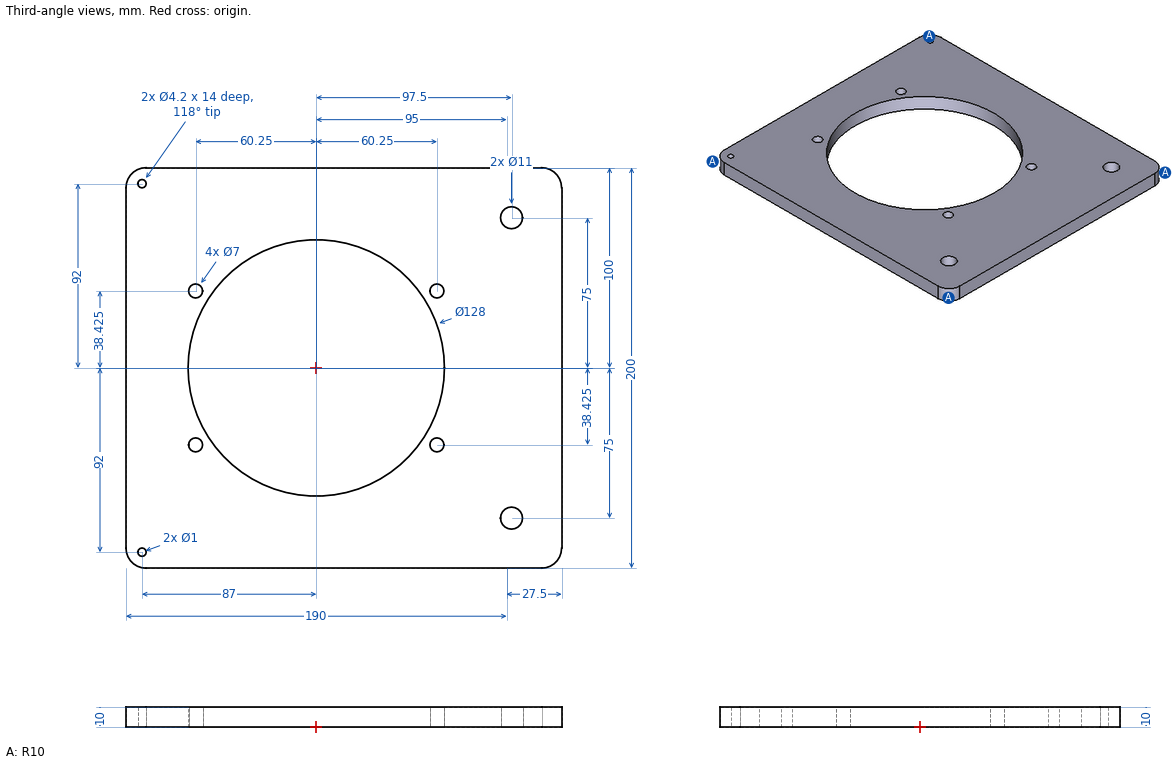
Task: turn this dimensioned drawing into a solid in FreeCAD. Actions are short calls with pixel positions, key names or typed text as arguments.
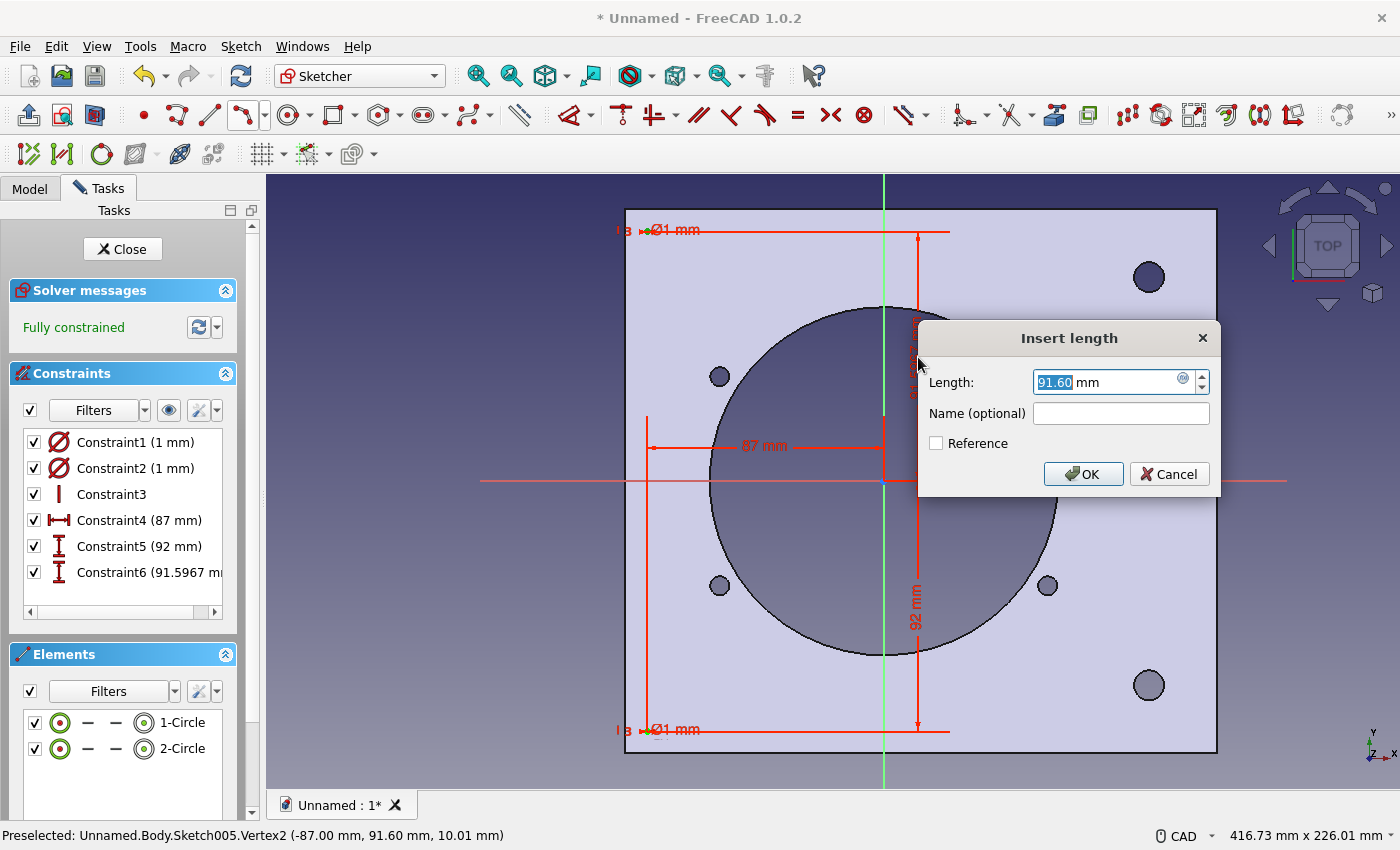
text(92)
key(Return)
key(Escape)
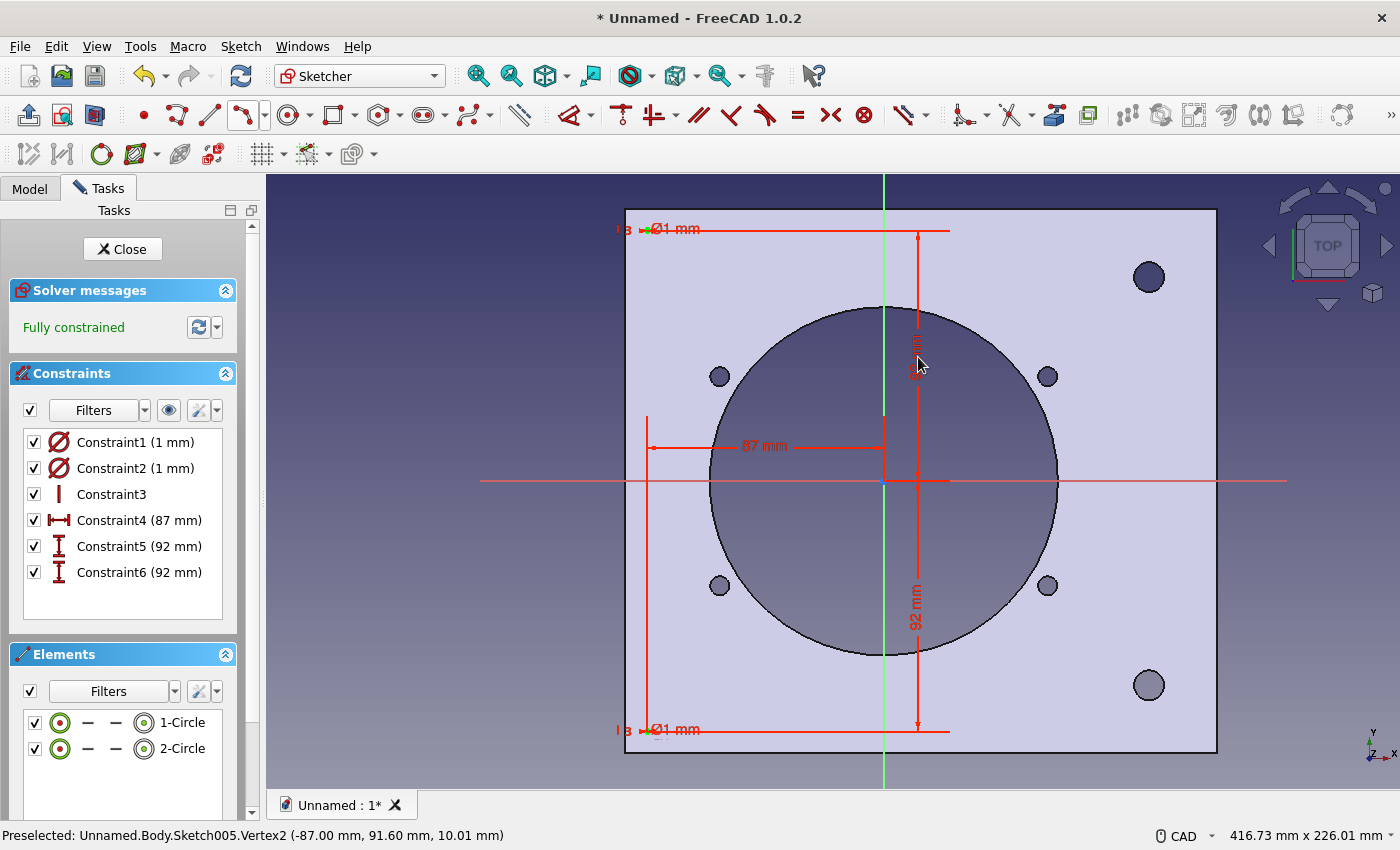
click(123, 249)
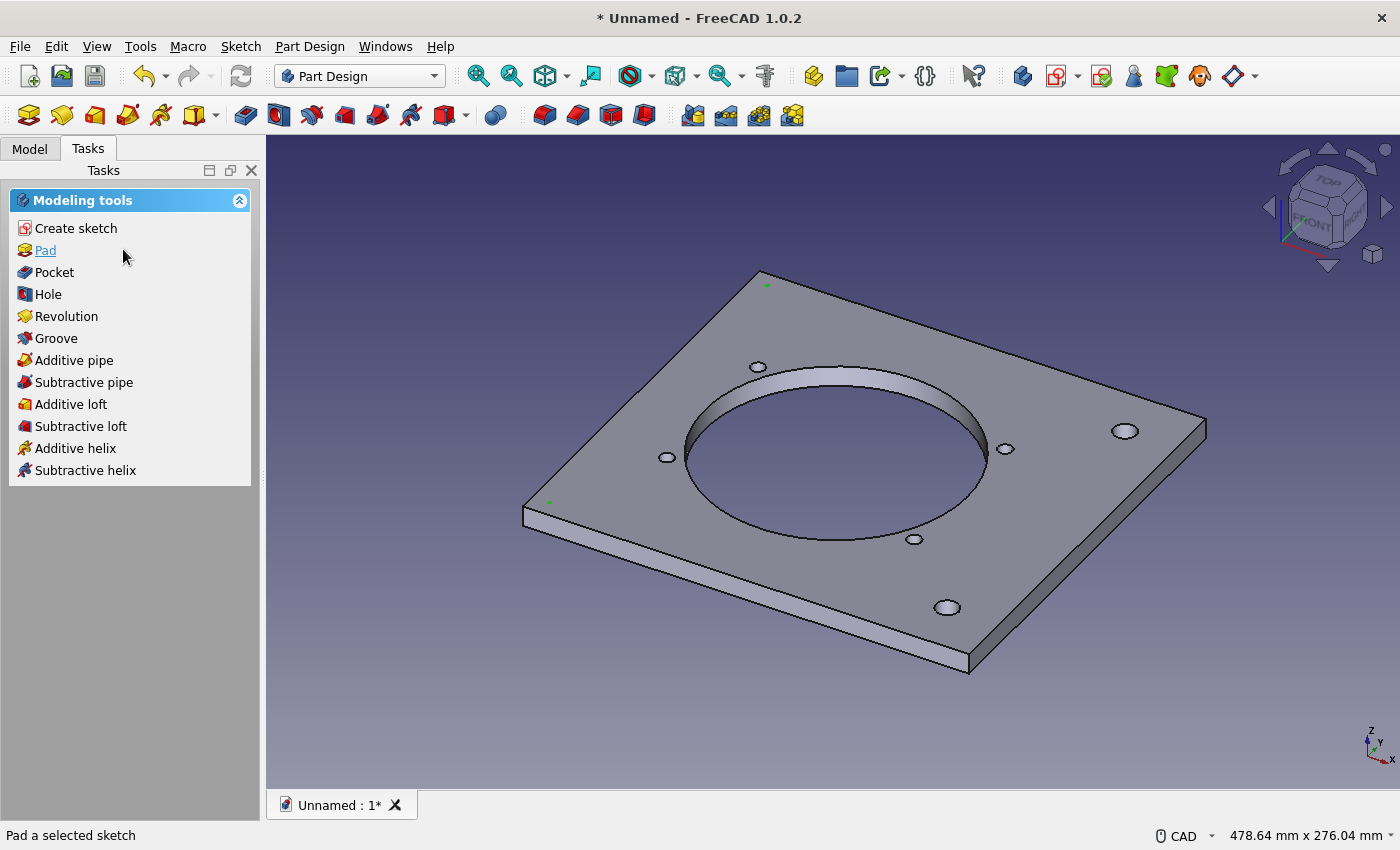
click(246, 116)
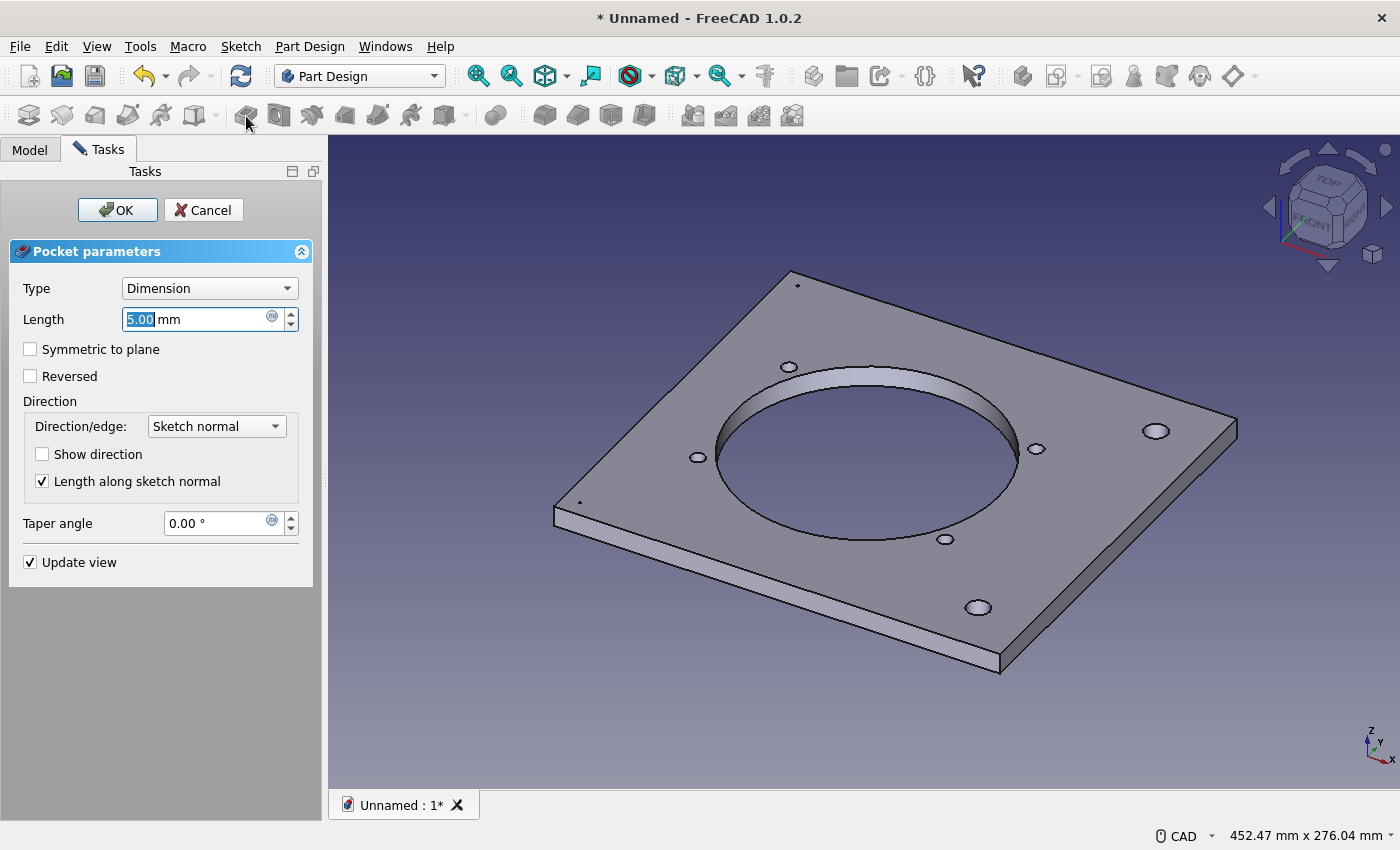
text(10)
key(Tab)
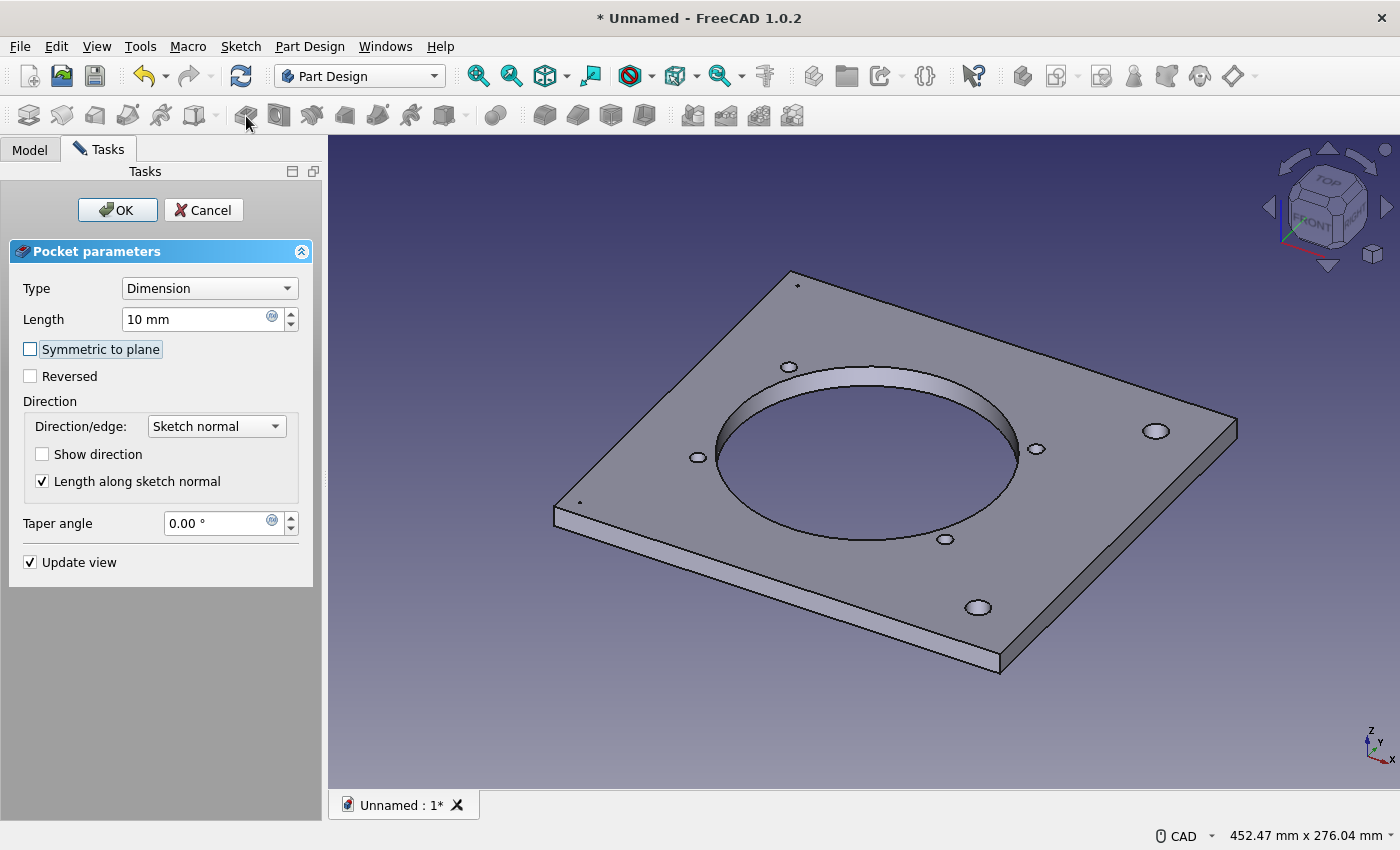
click(118, 210)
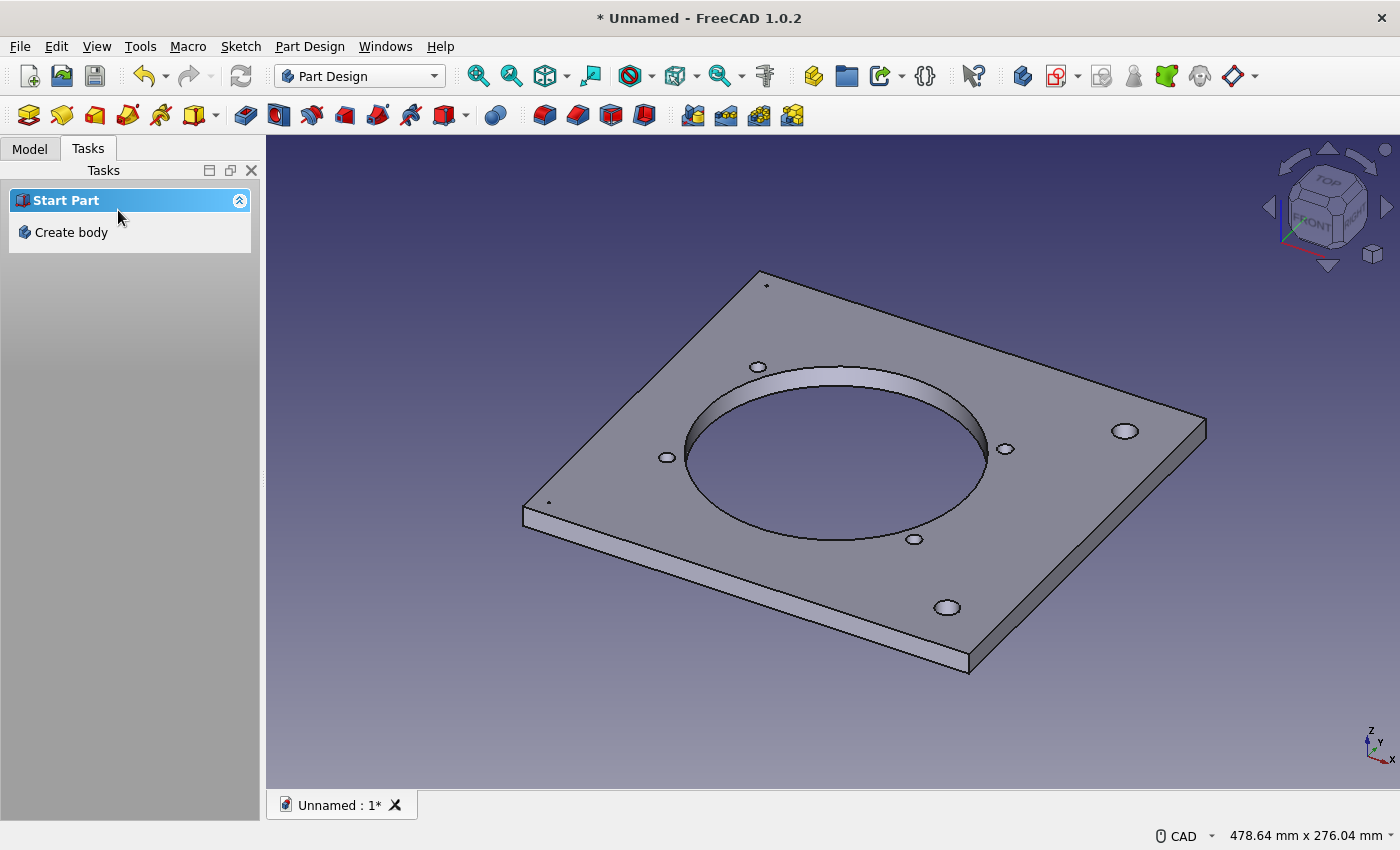
click(924, 571)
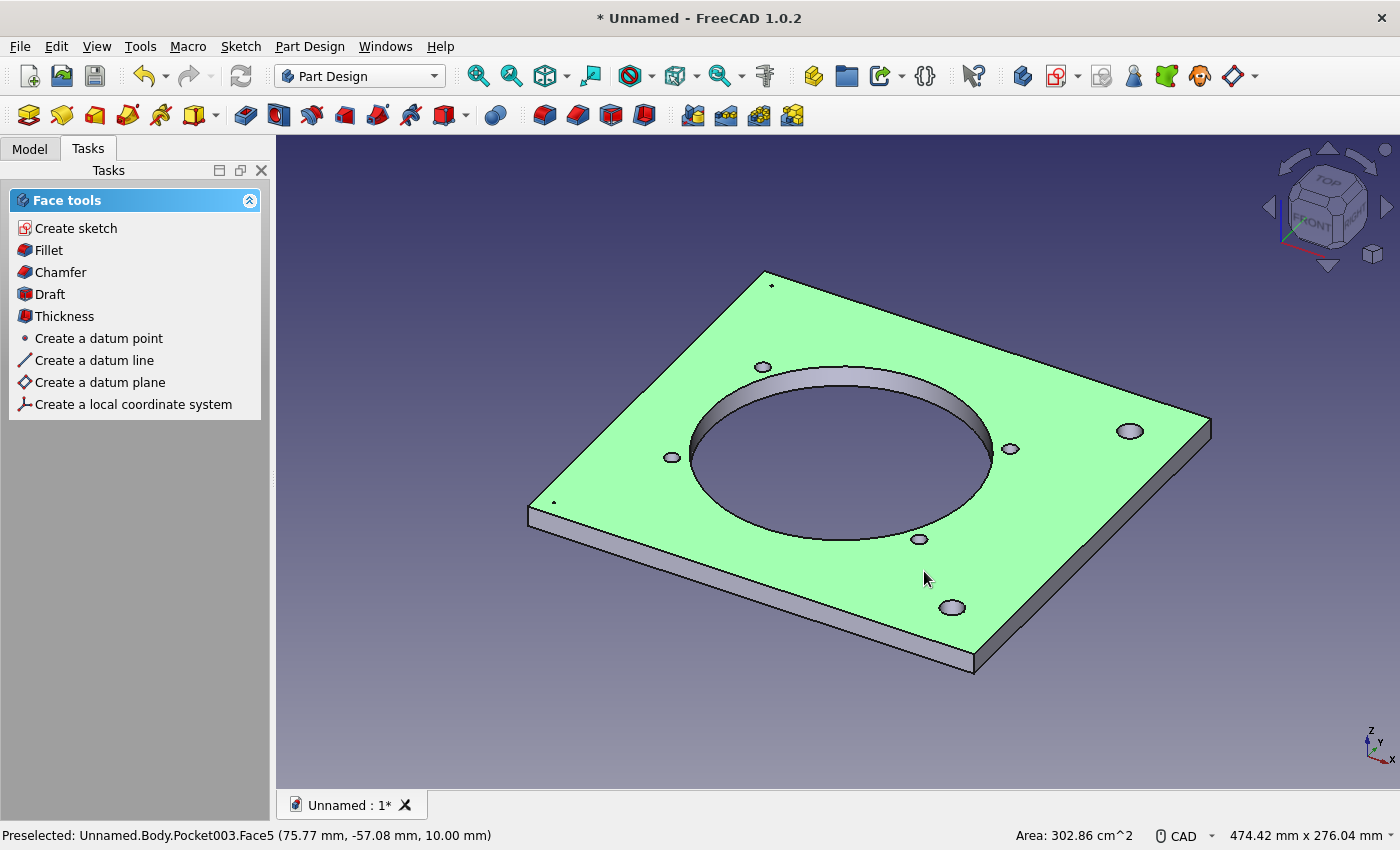
click(1056, 76)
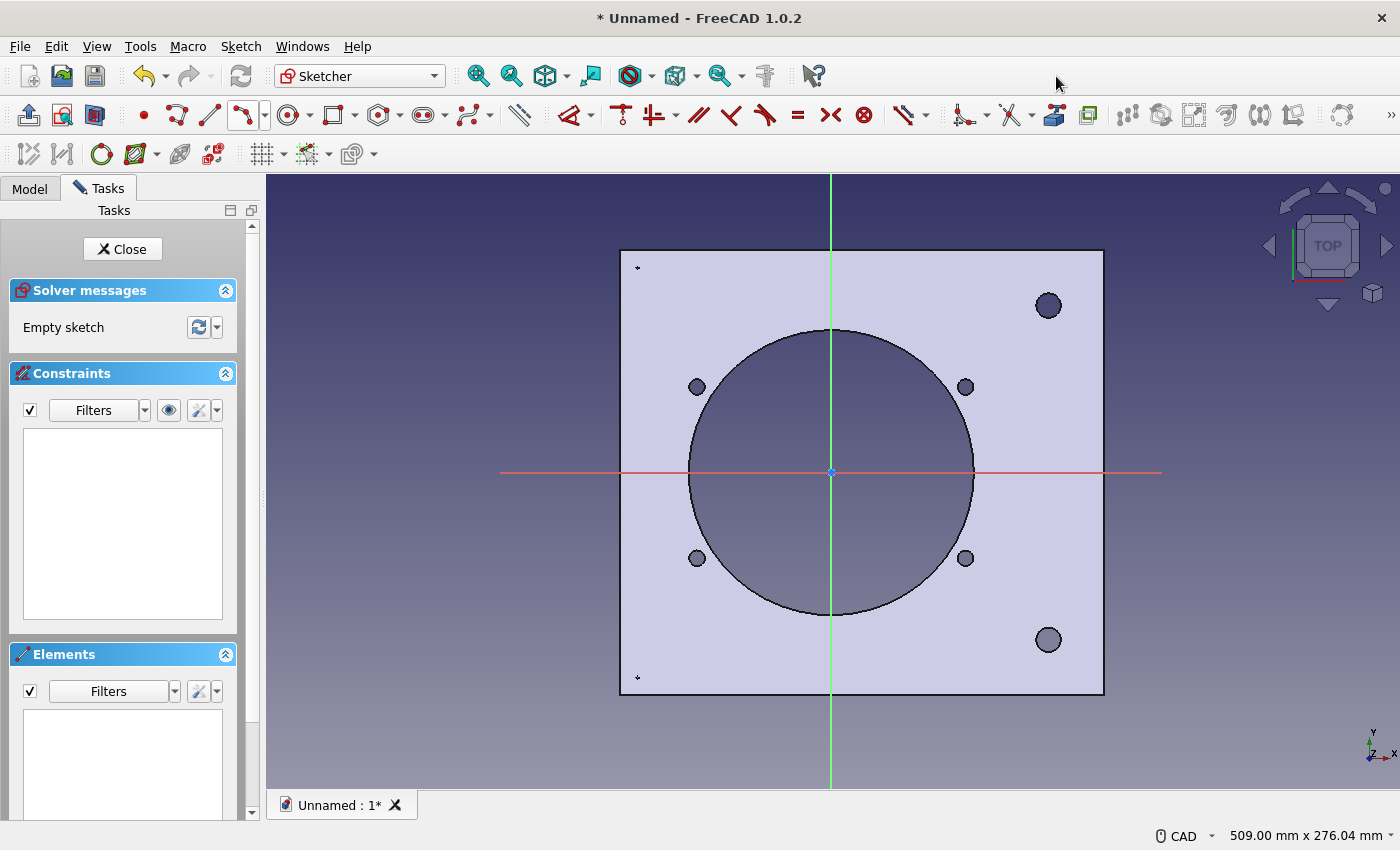
key(g)
key(c)